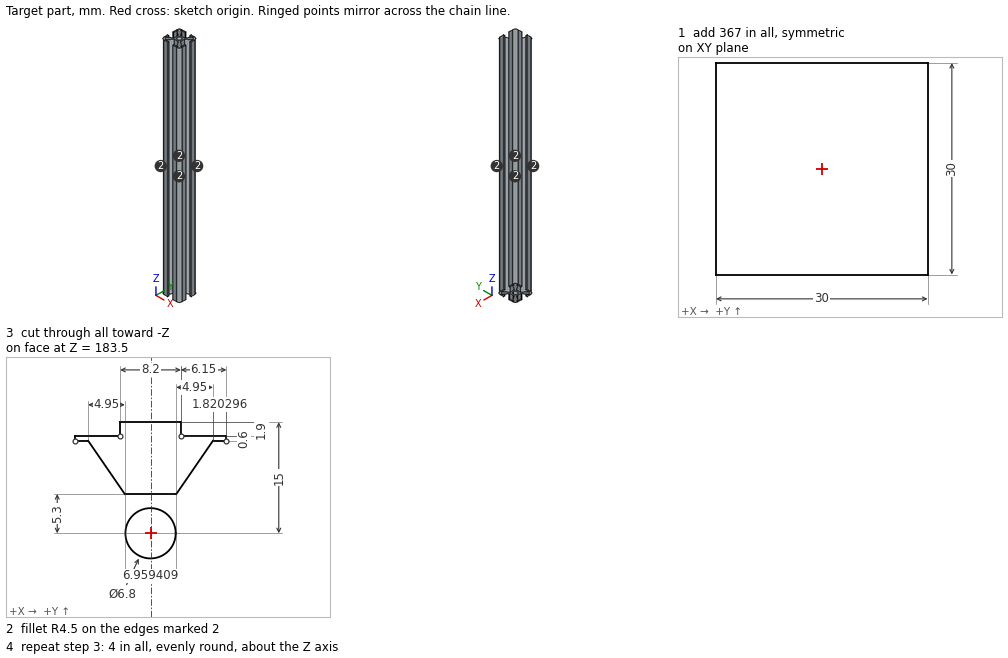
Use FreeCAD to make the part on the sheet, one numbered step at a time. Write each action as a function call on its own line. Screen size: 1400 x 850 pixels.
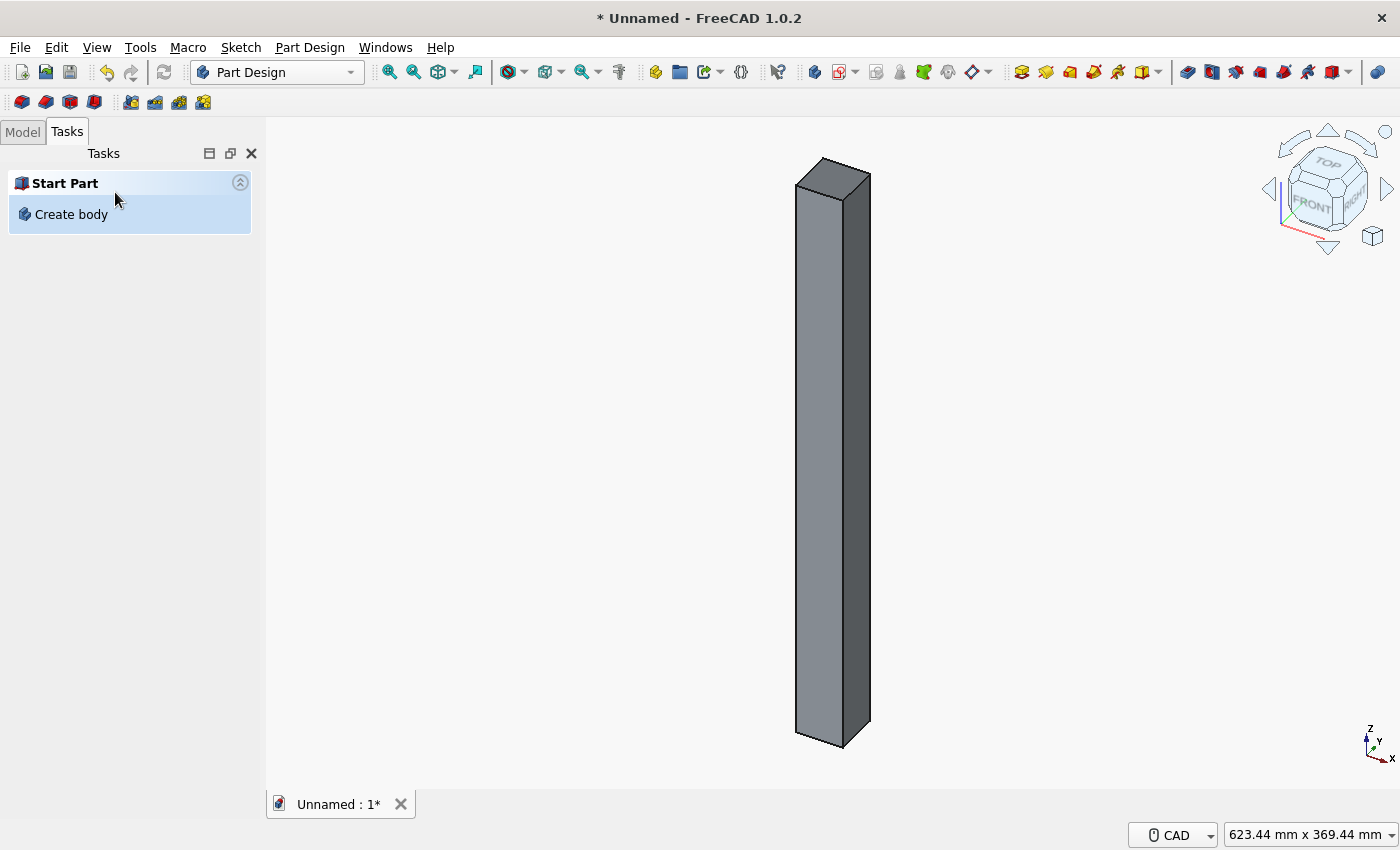
click(843, 473)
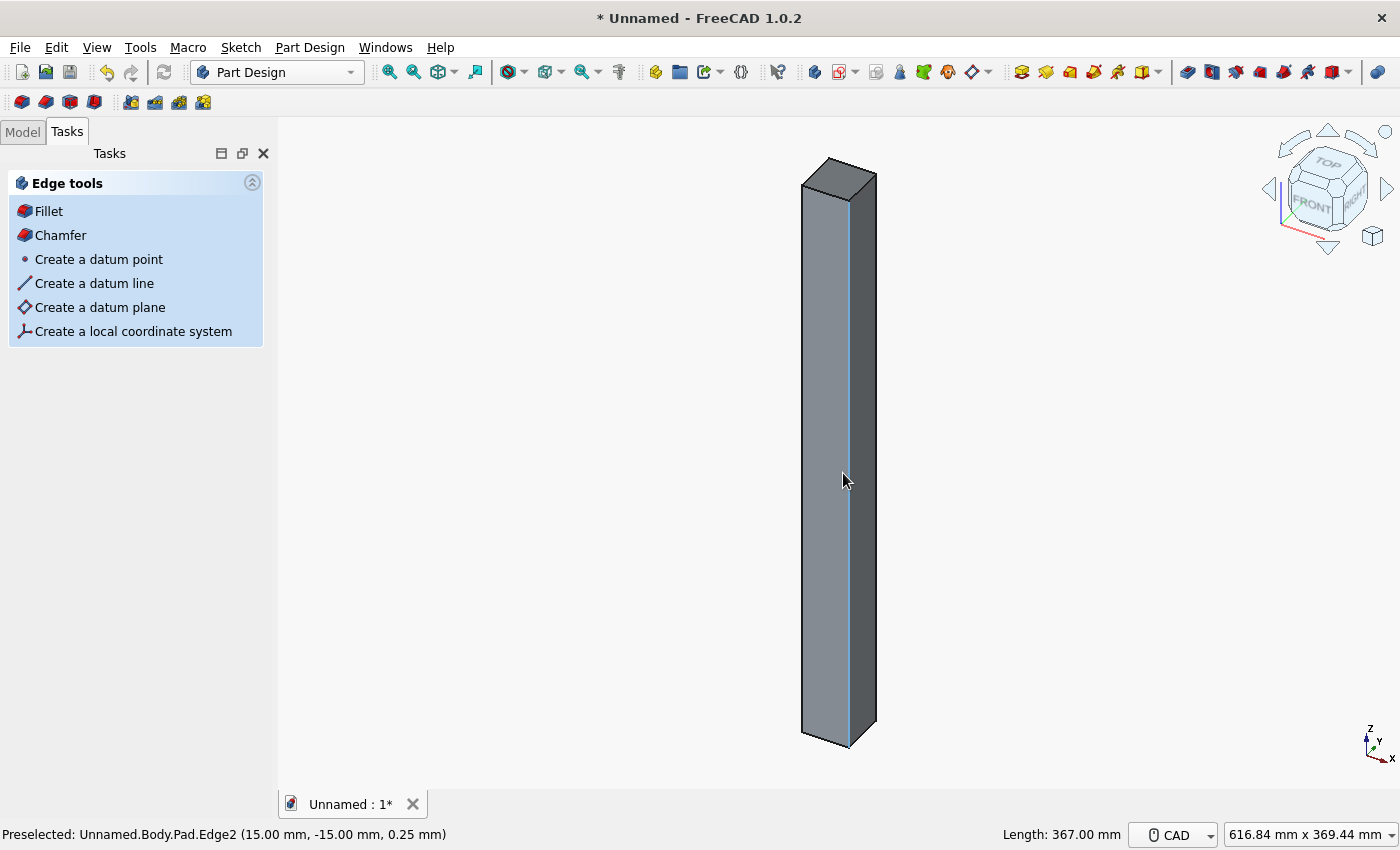
key(0)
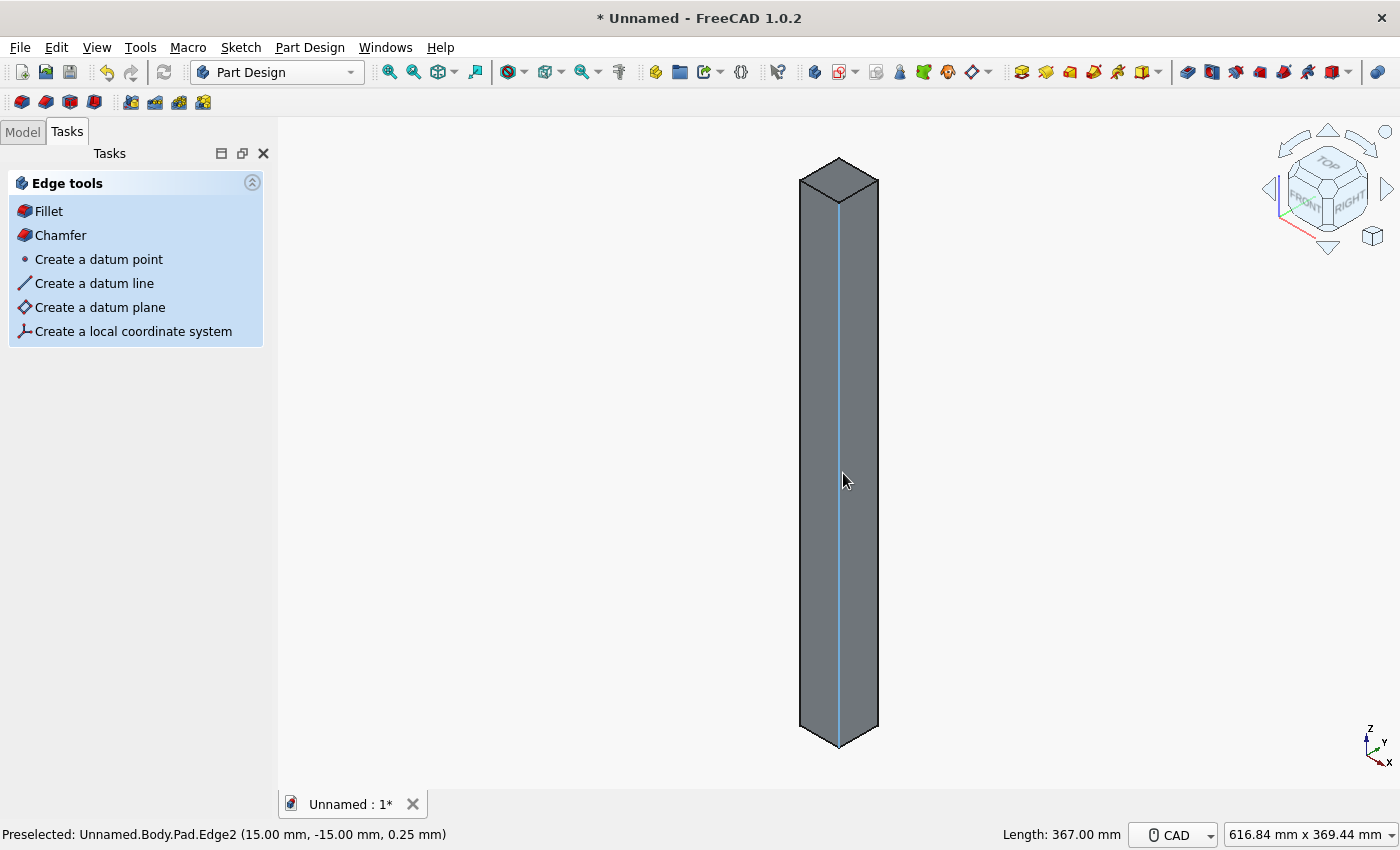
key(2)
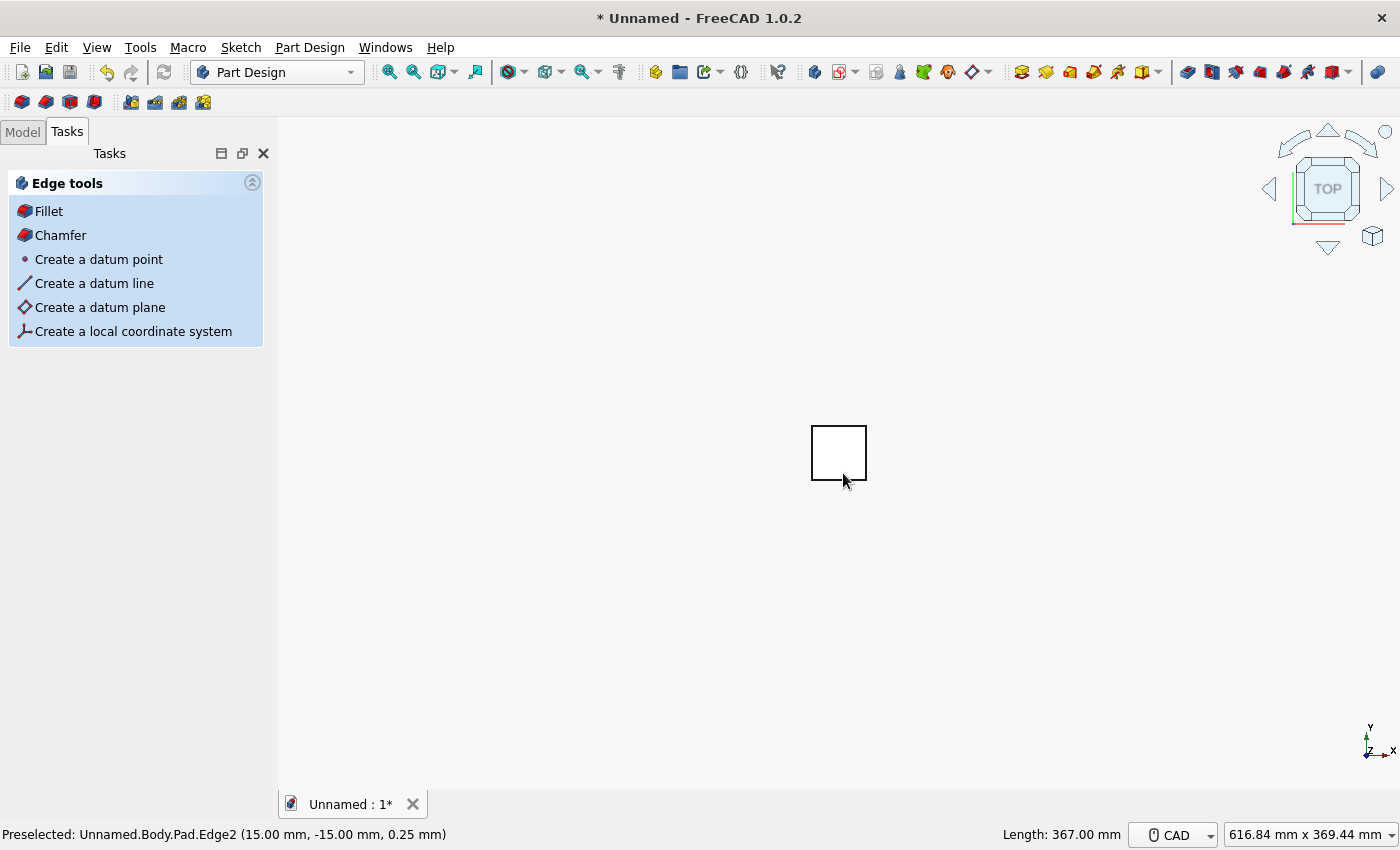
key(v)
key(f)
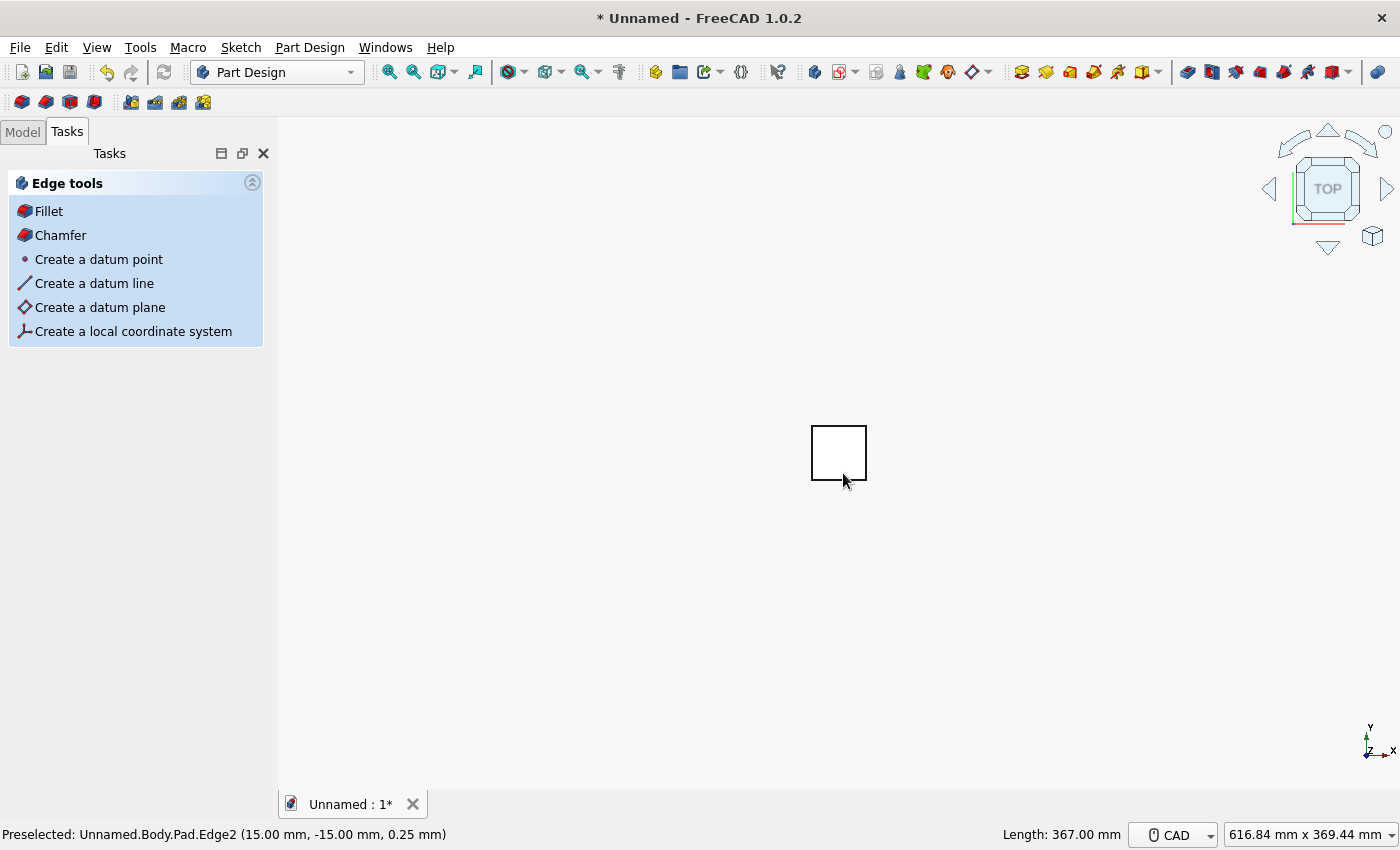
key(1)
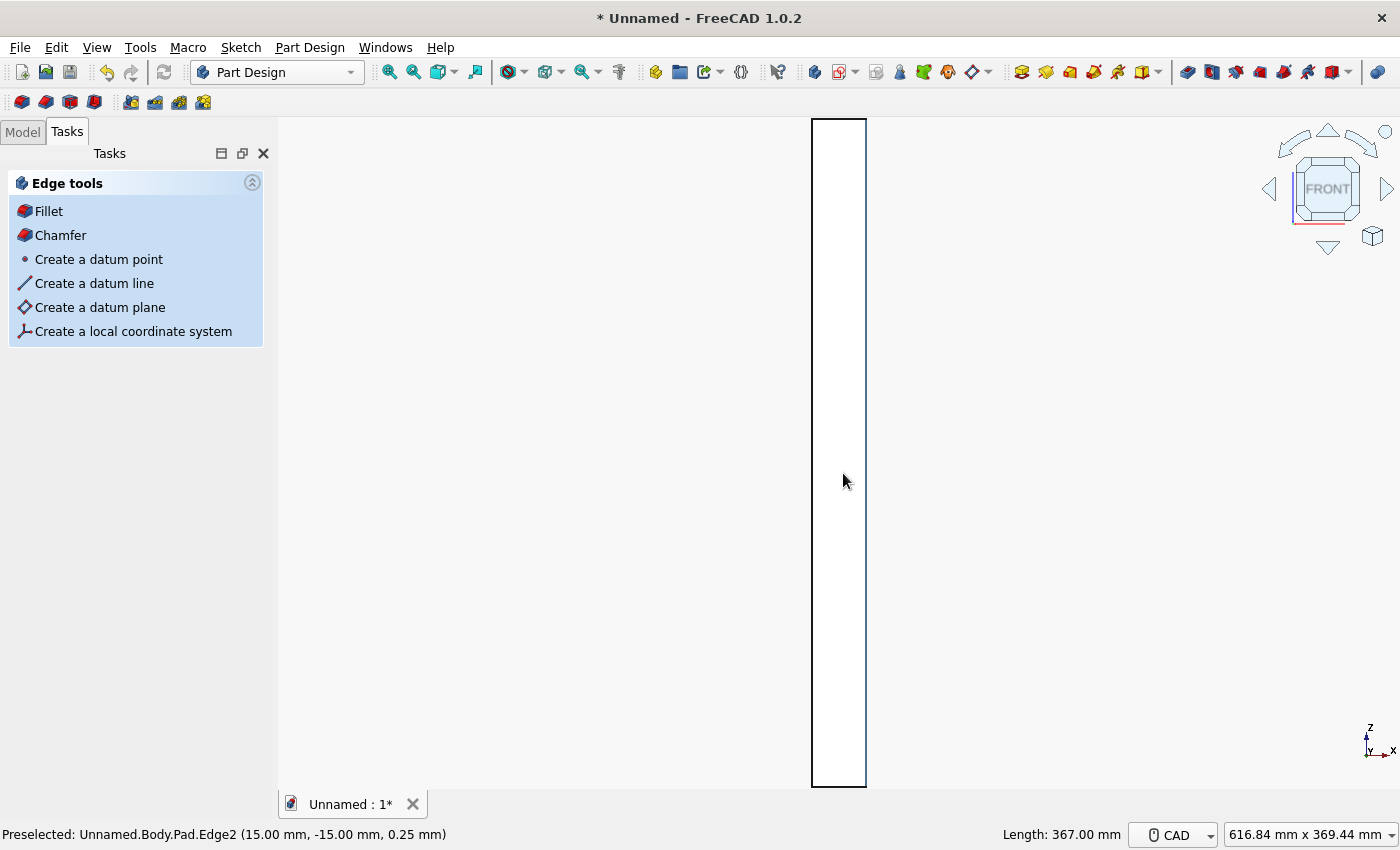
click(812, 452, ctrl)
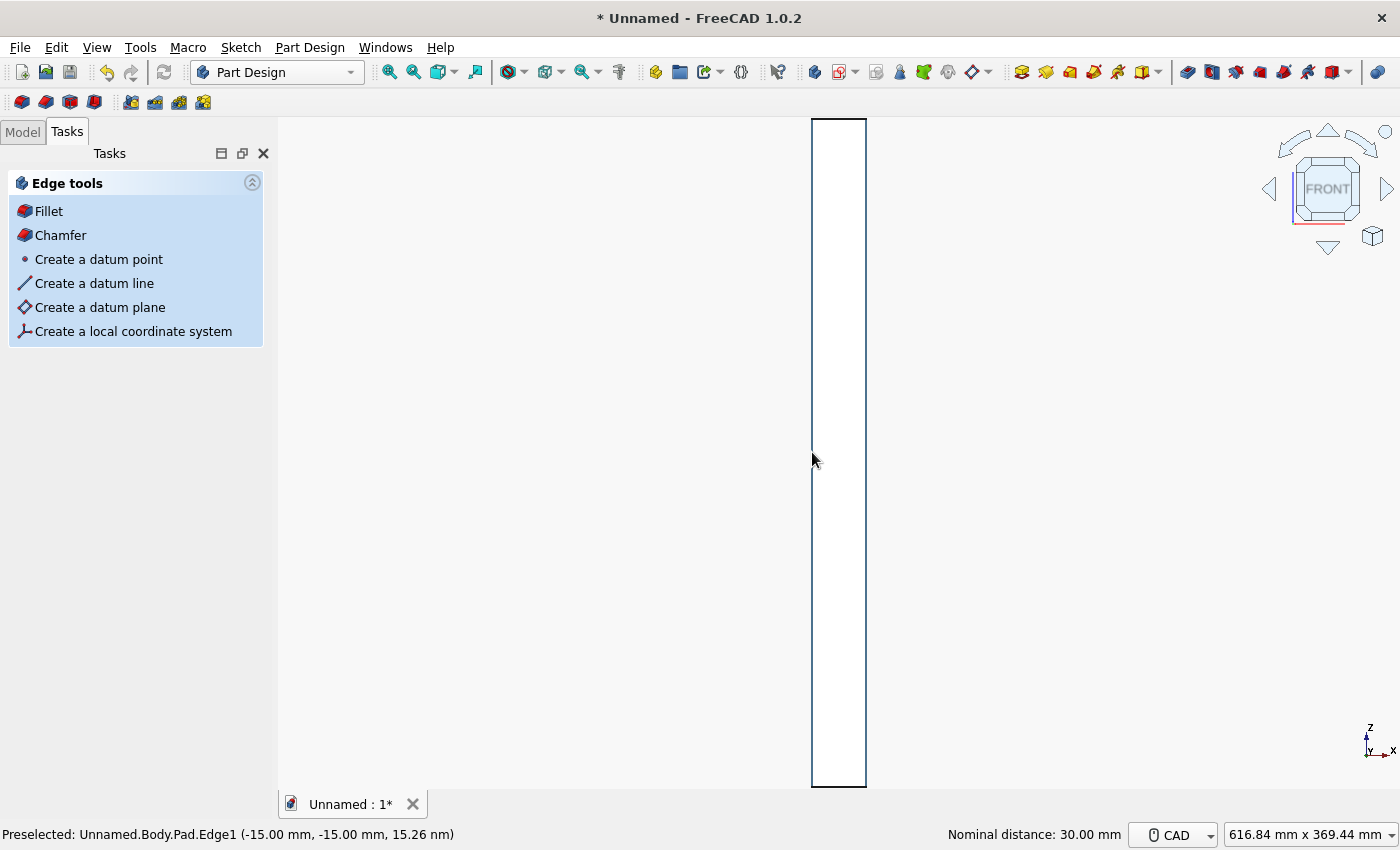
key(3)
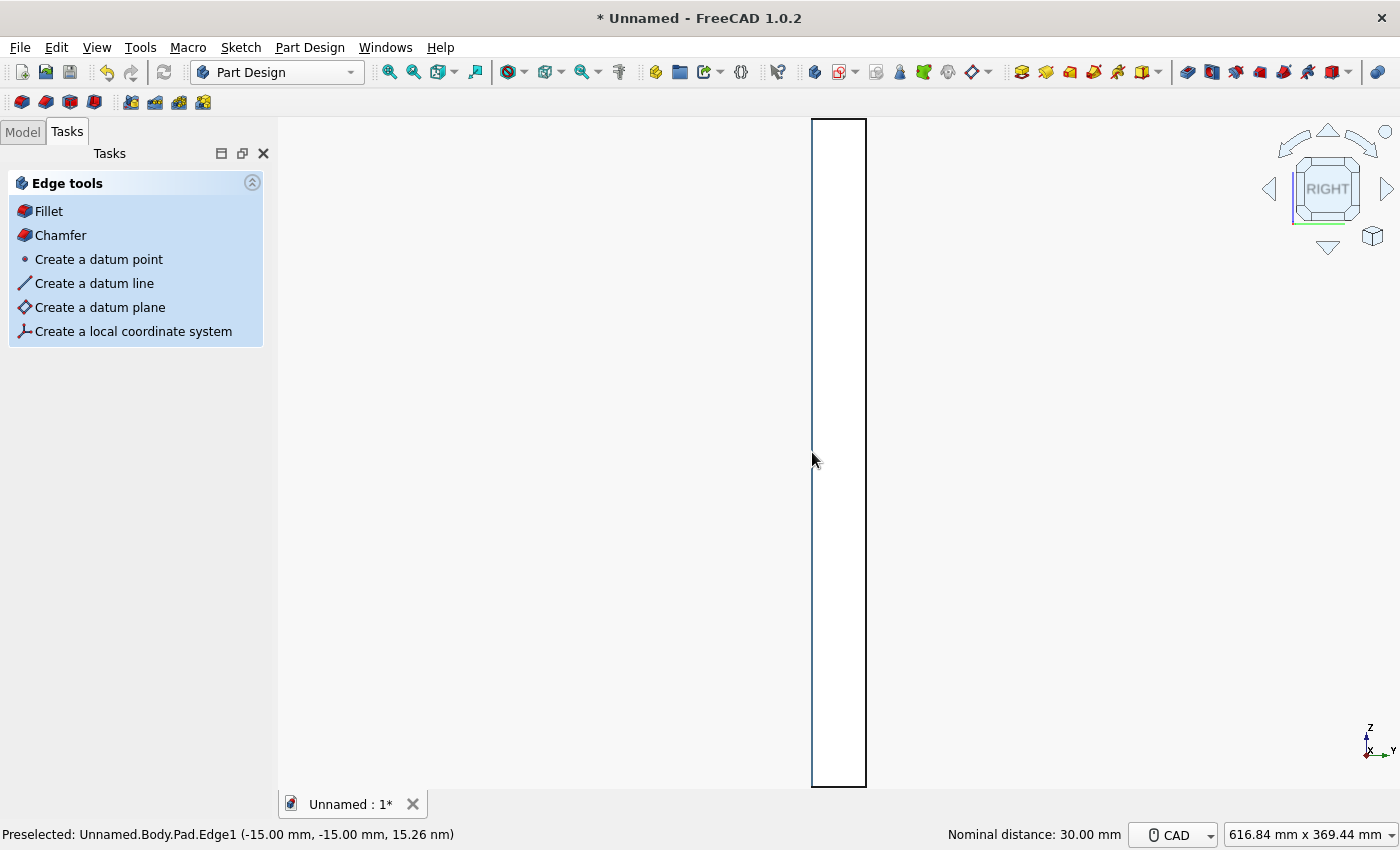
click(866, 452, ctrl)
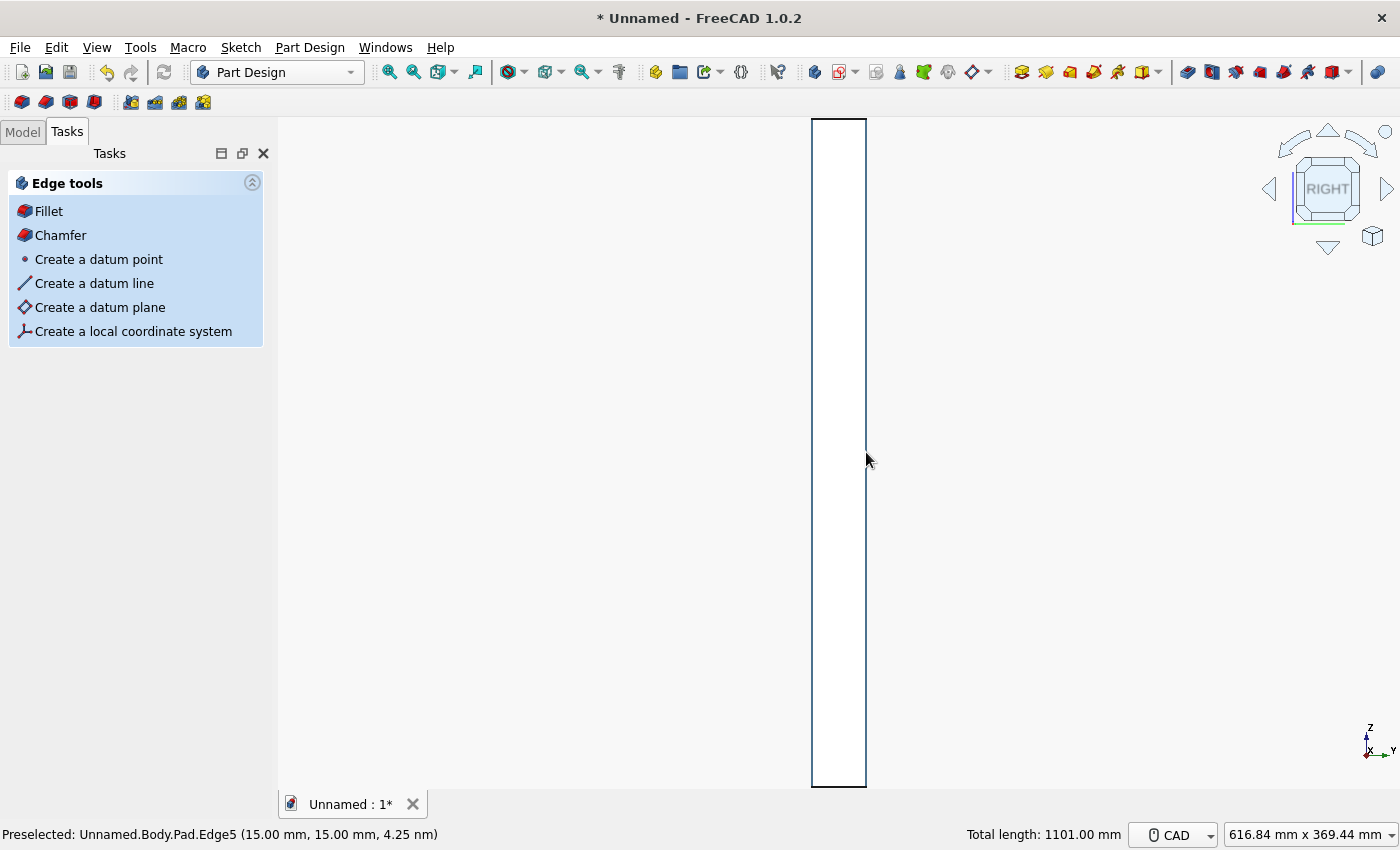
key(5)